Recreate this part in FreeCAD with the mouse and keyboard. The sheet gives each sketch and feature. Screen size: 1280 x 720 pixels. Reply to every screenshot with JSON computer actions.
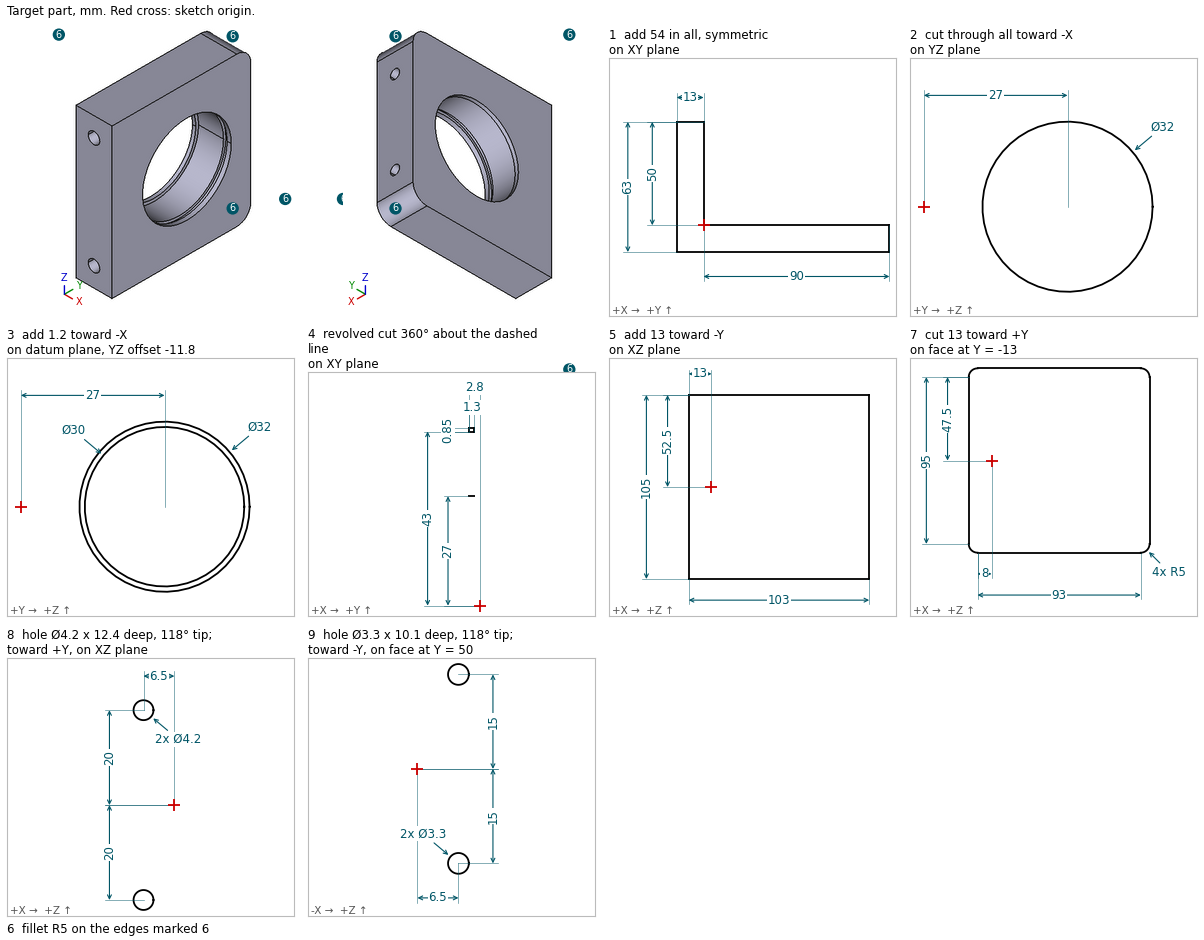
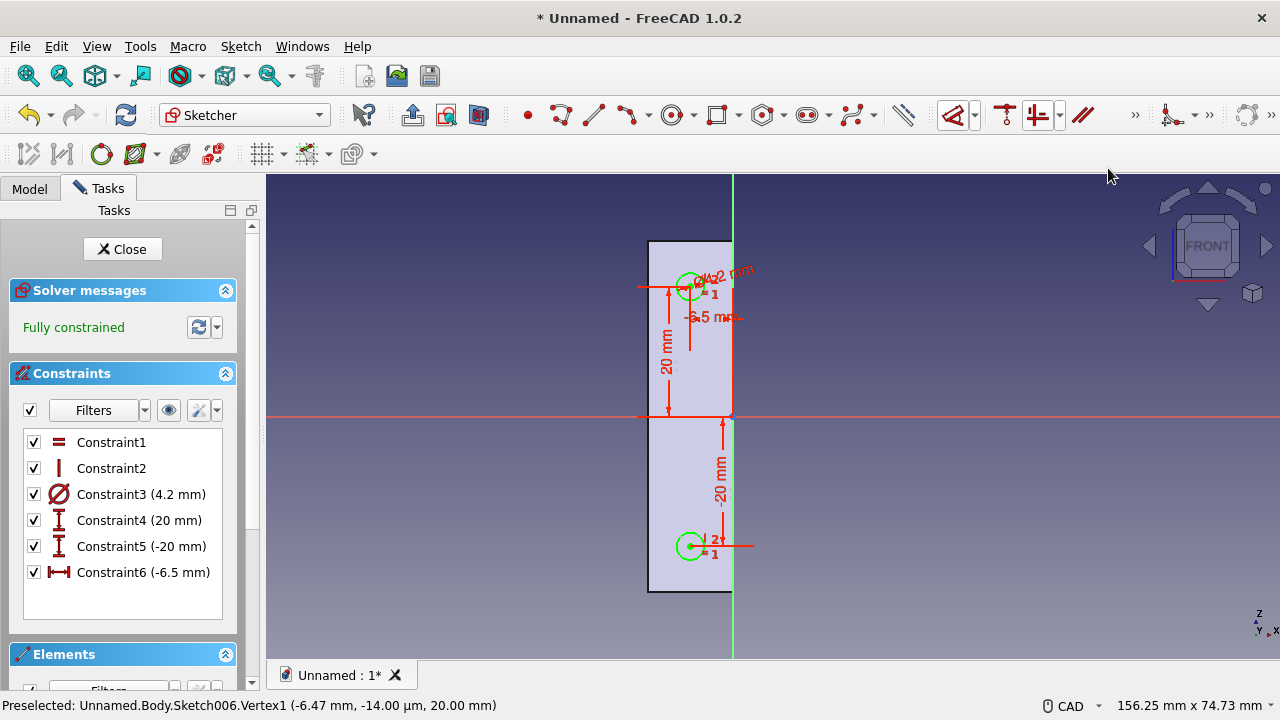
{"action": "left_click", "coordinate": [123, 249]}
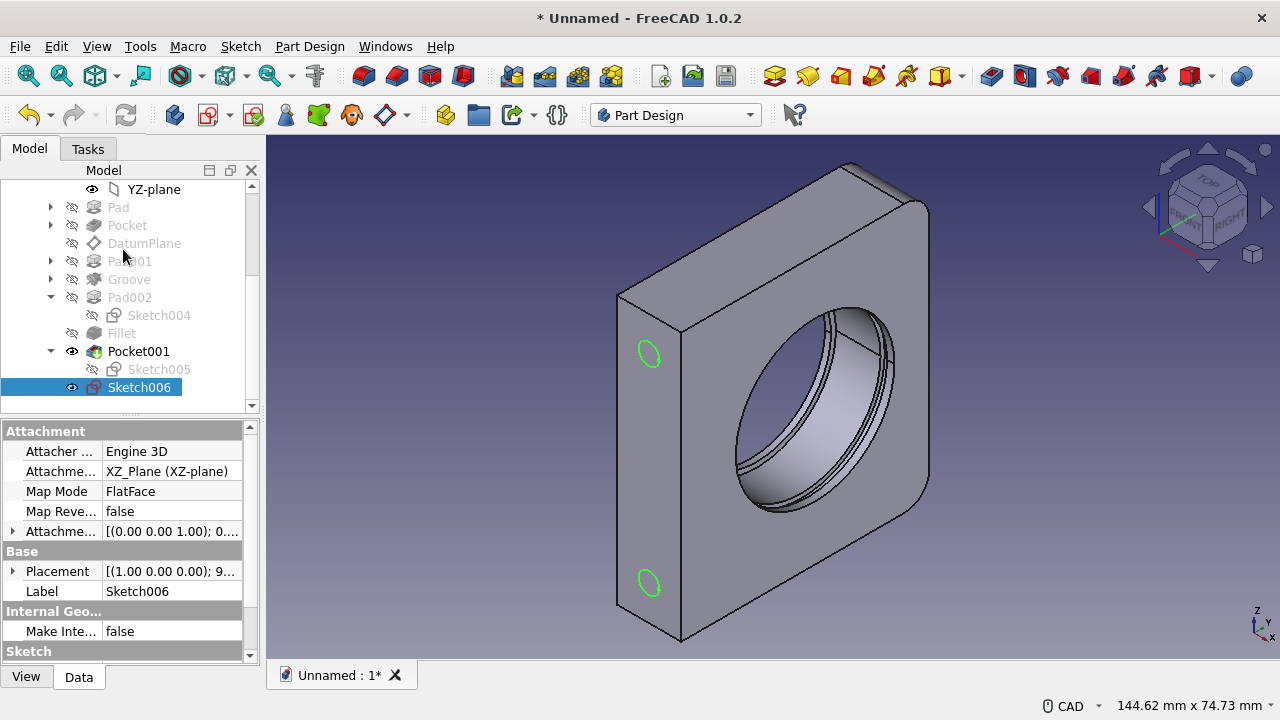
{"action": "left_click", "coordinate": [1025, 76]}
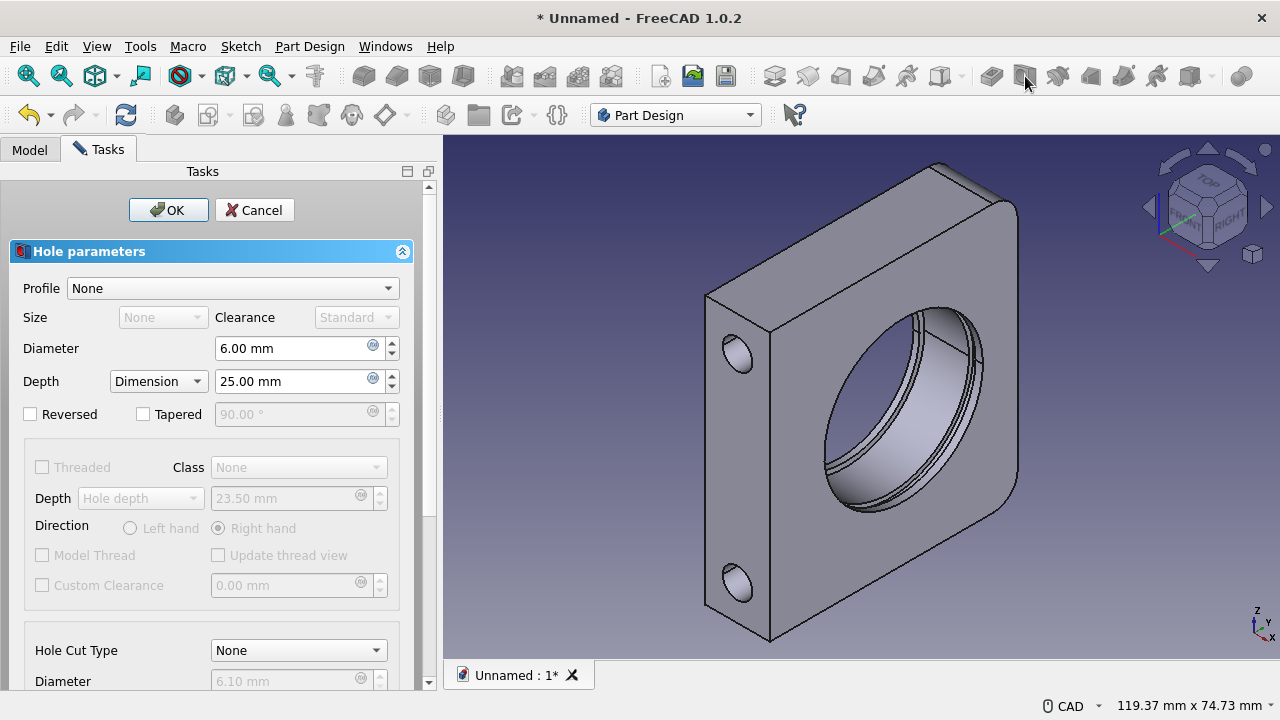
{"action": "triple_click", "coordinate": [300, 348]}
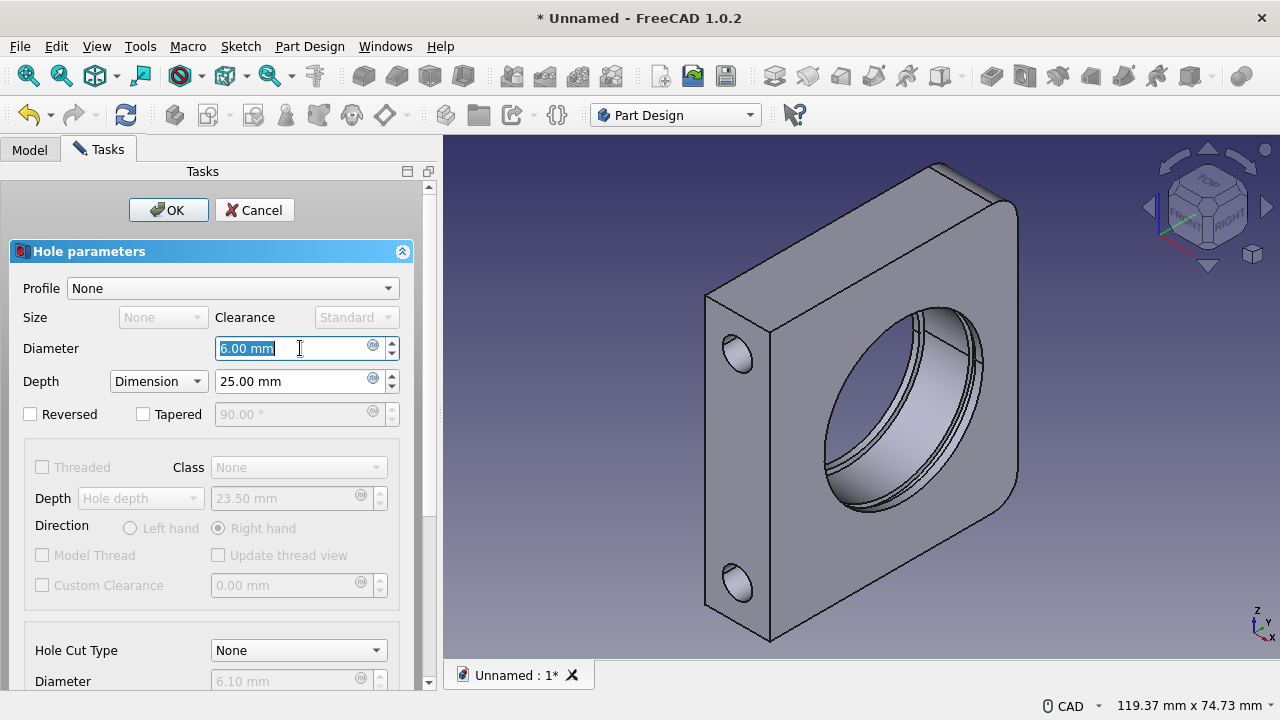
{"action": "type", "text": "4.2"}
{"action": "key", "text": "Tab"}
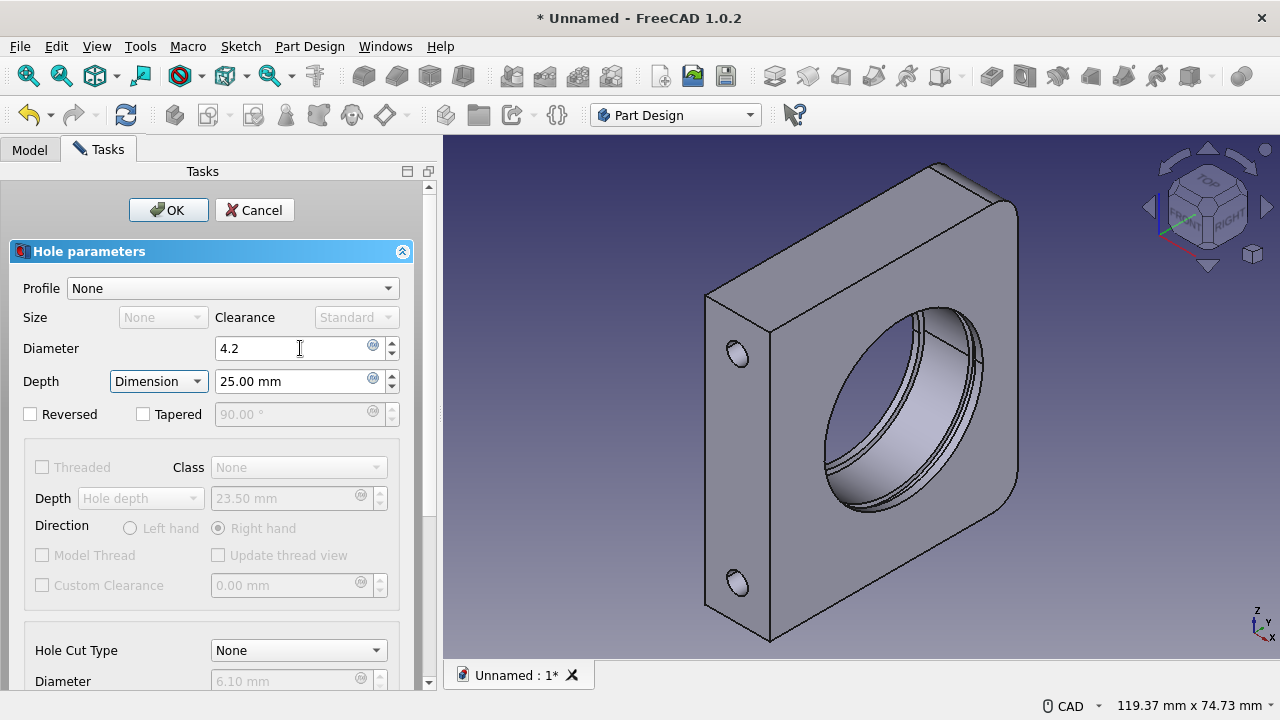
{"action": "triple_click", "coordinate": [300, 382]}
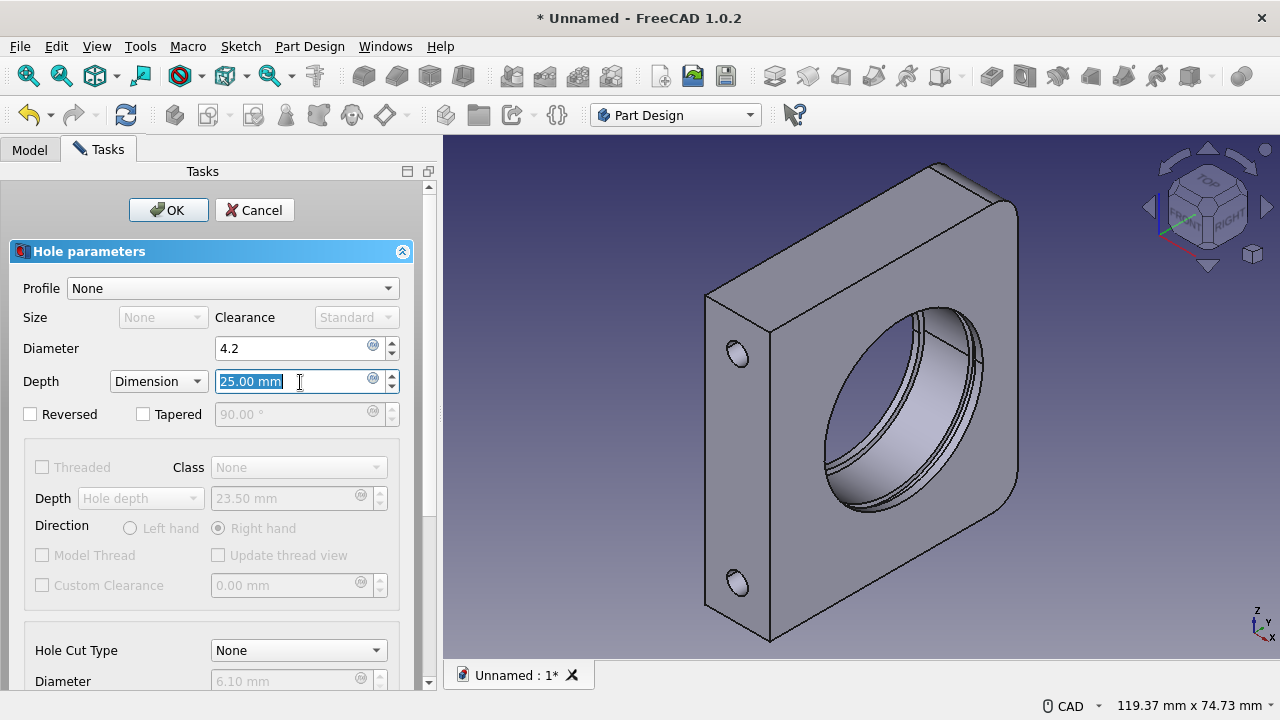
{"action": "type", "text": "12.4"}
{"action": "key", "text": "Tab"}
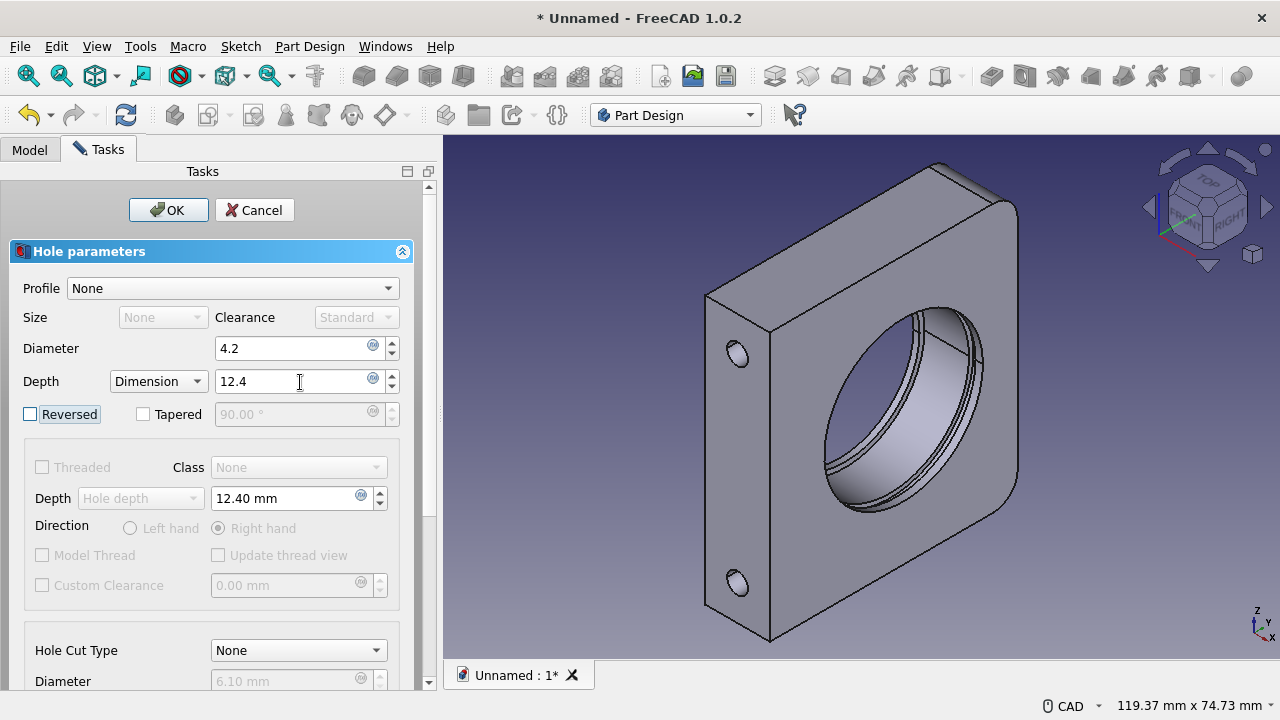
{"action": "left_click", "coordinate": [169, 210]}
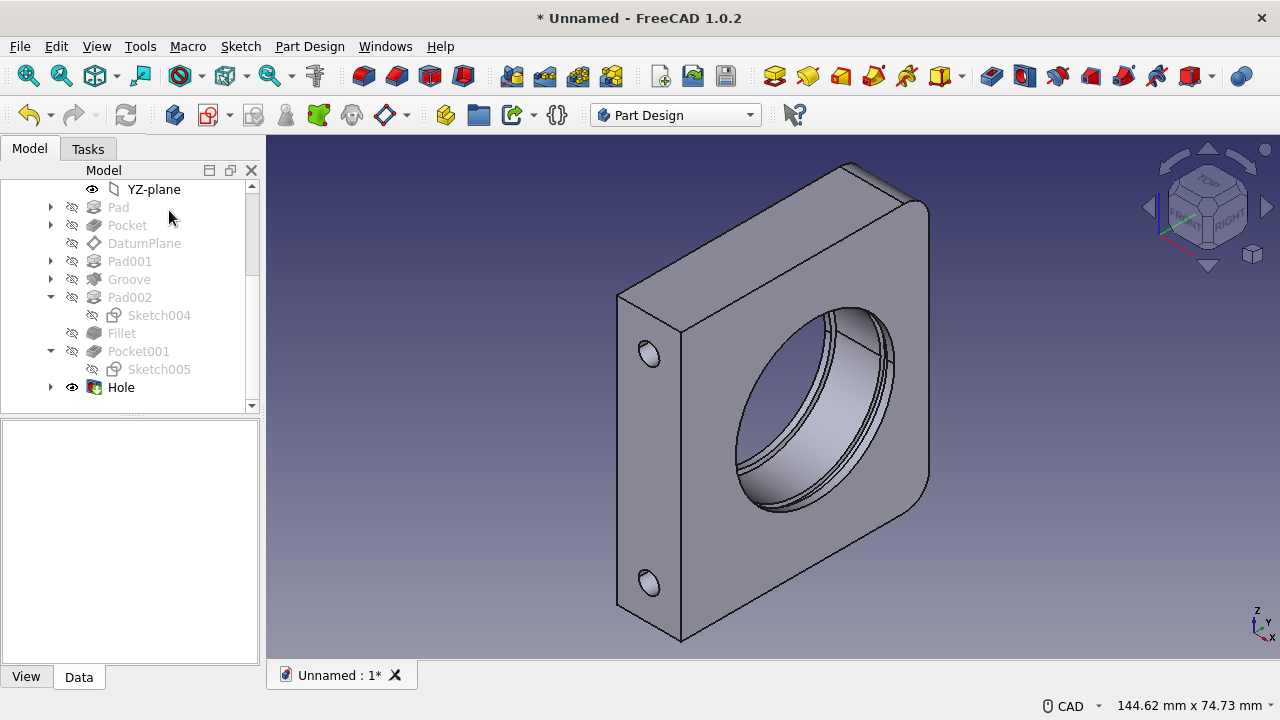
{"action": "key", "text": "4"}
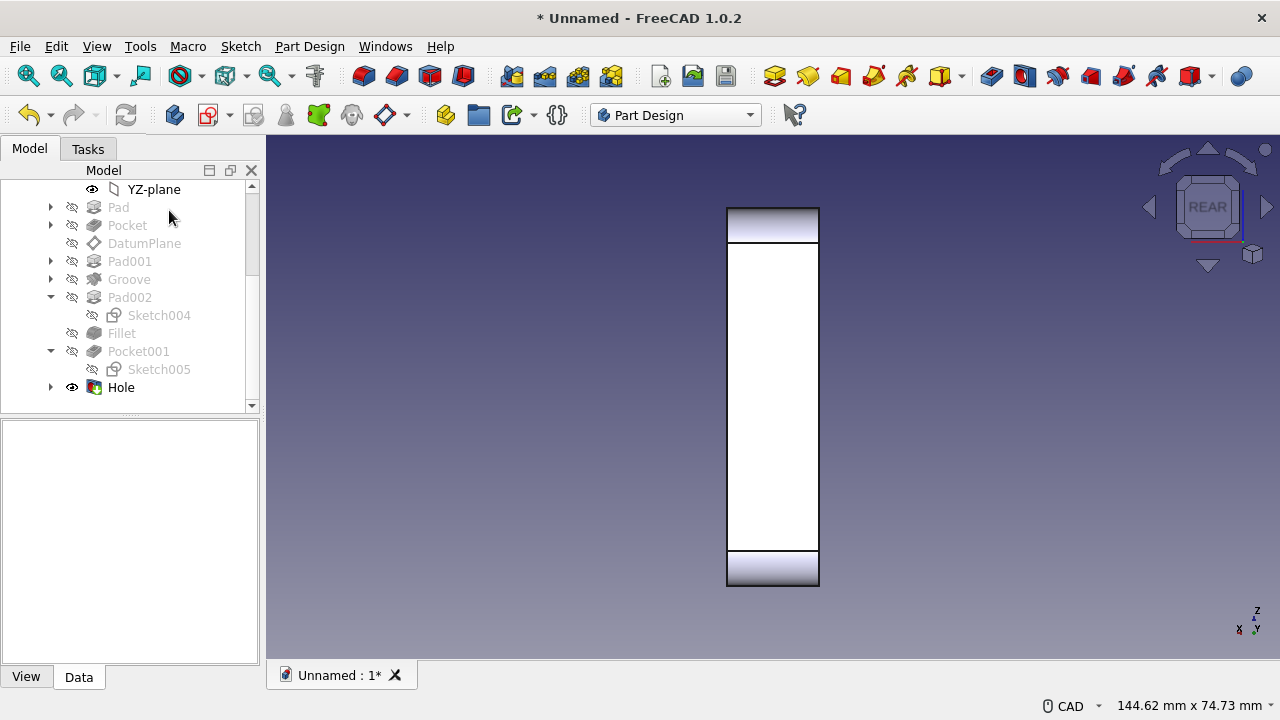
{"action": "left_click", "coordinate": [773, 308]}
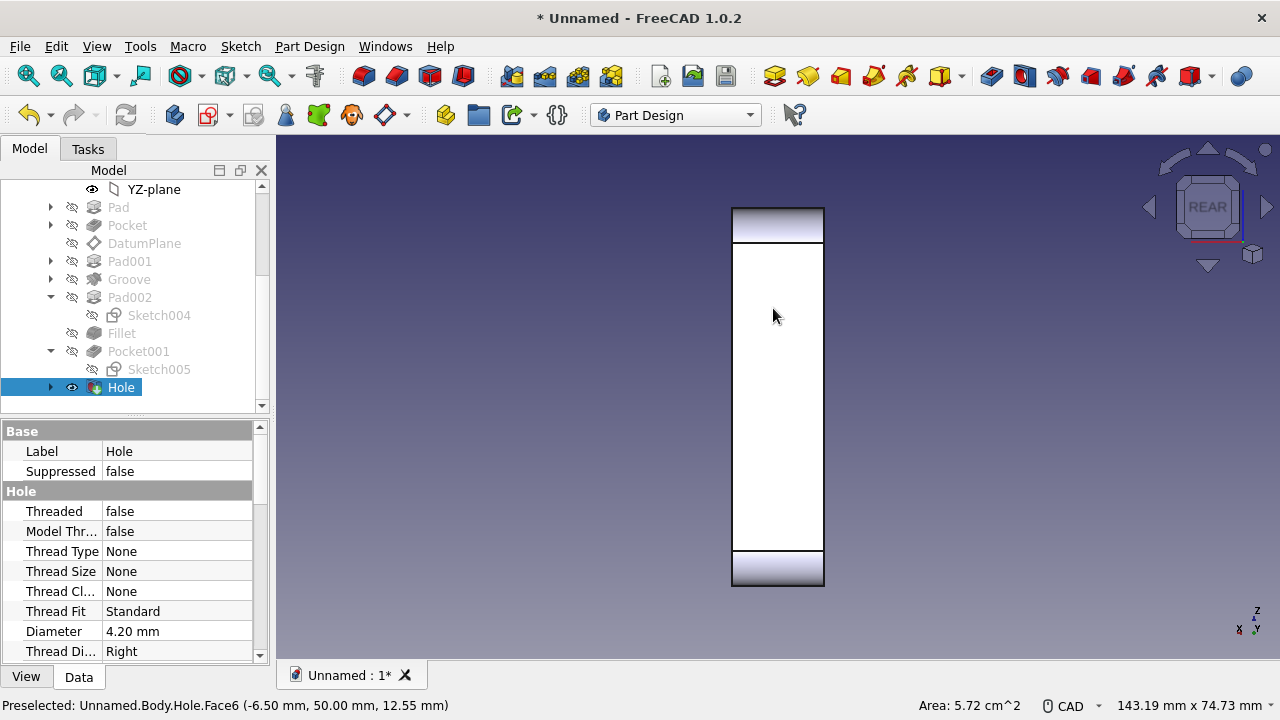
{"action": "left_click", "coordinate": [208, 116]}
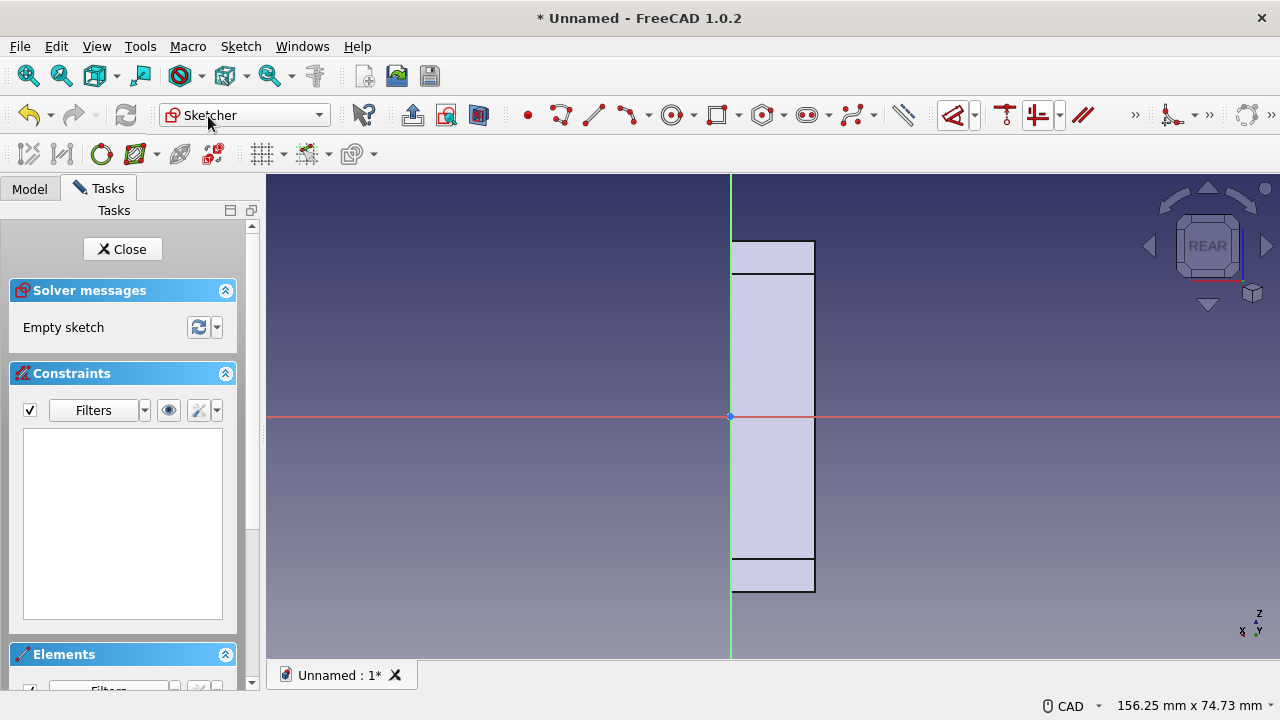
{"action": "scroll", "coordinate": [865, 416], "scroll_direction": "up", "scroll_amount": 2}